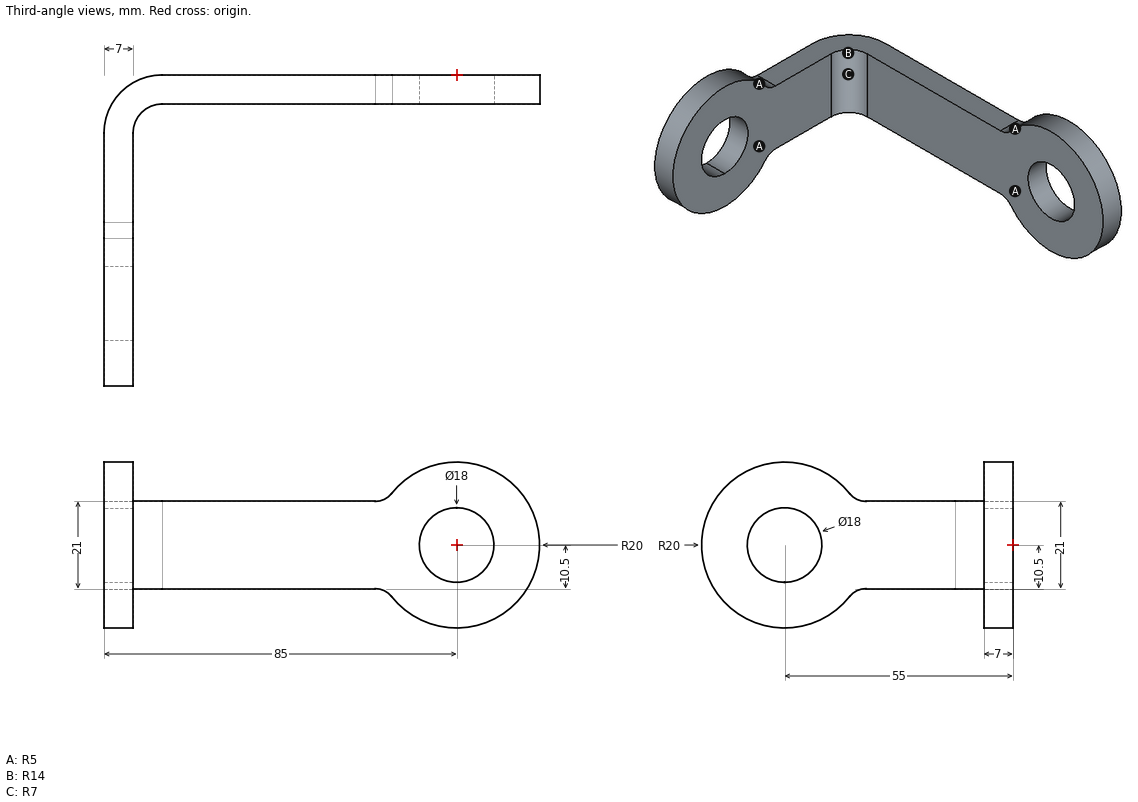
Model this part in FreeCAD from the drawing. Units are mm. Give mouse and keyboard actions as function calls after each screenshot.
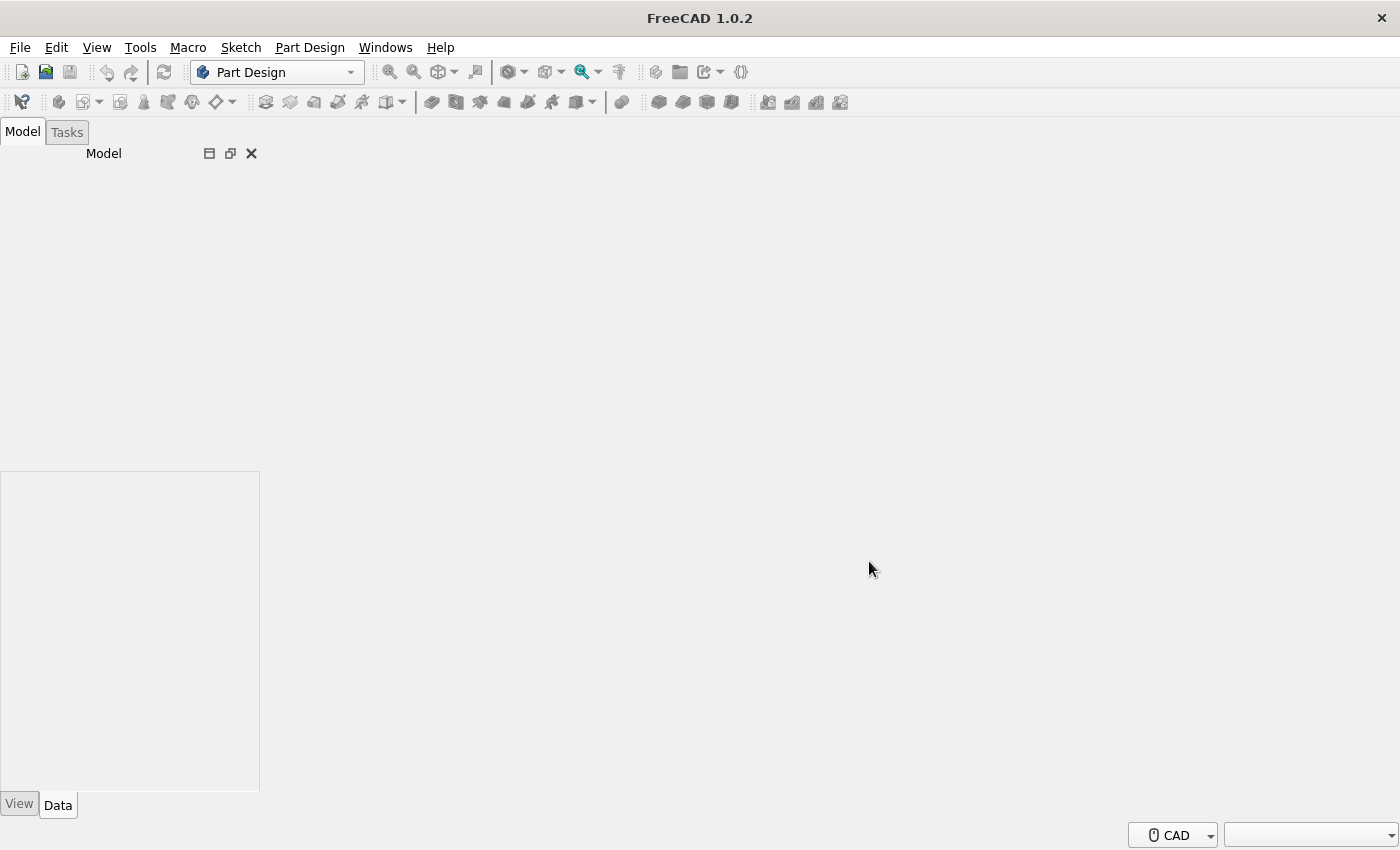
click(22, 72)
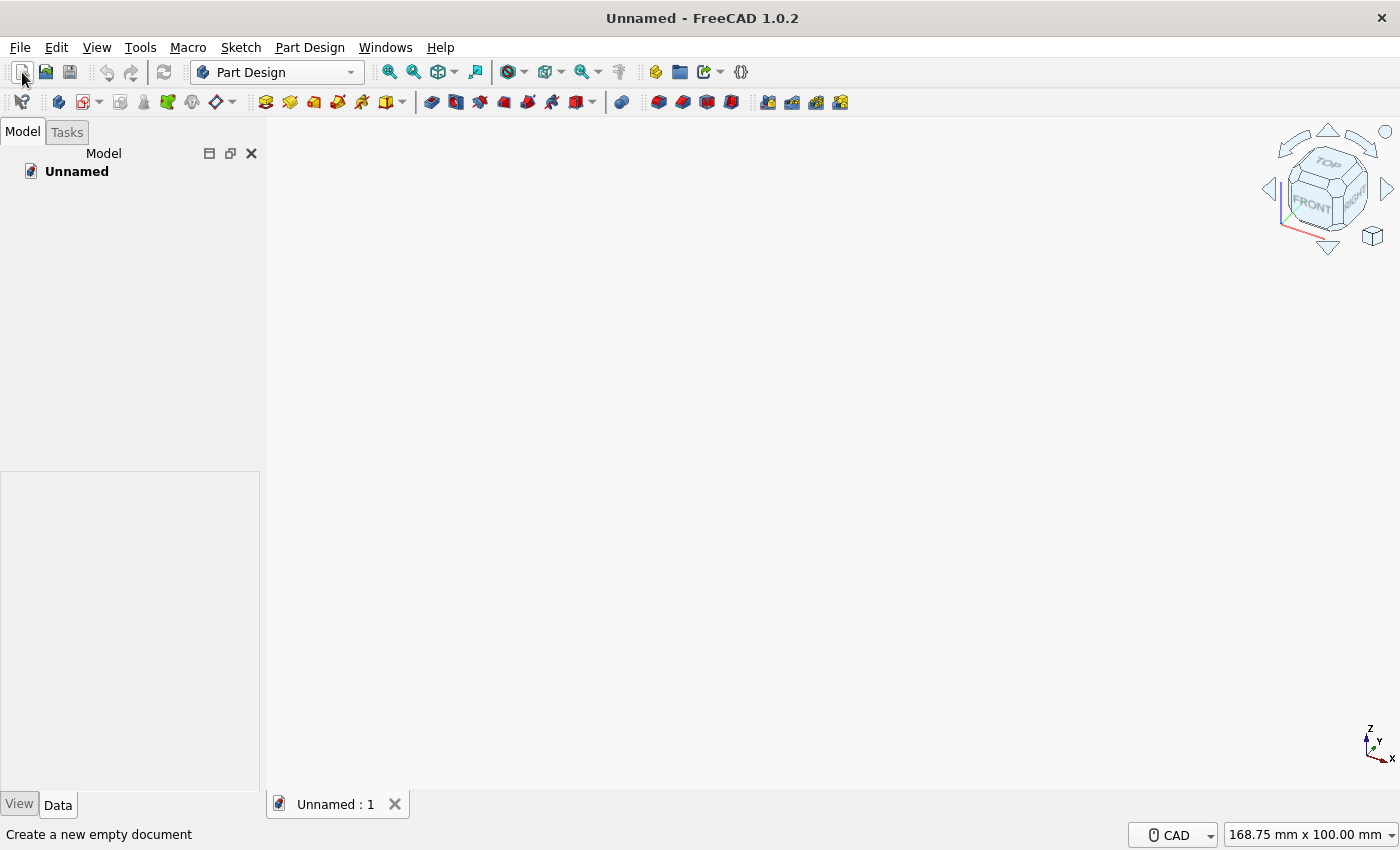
click(84, 102)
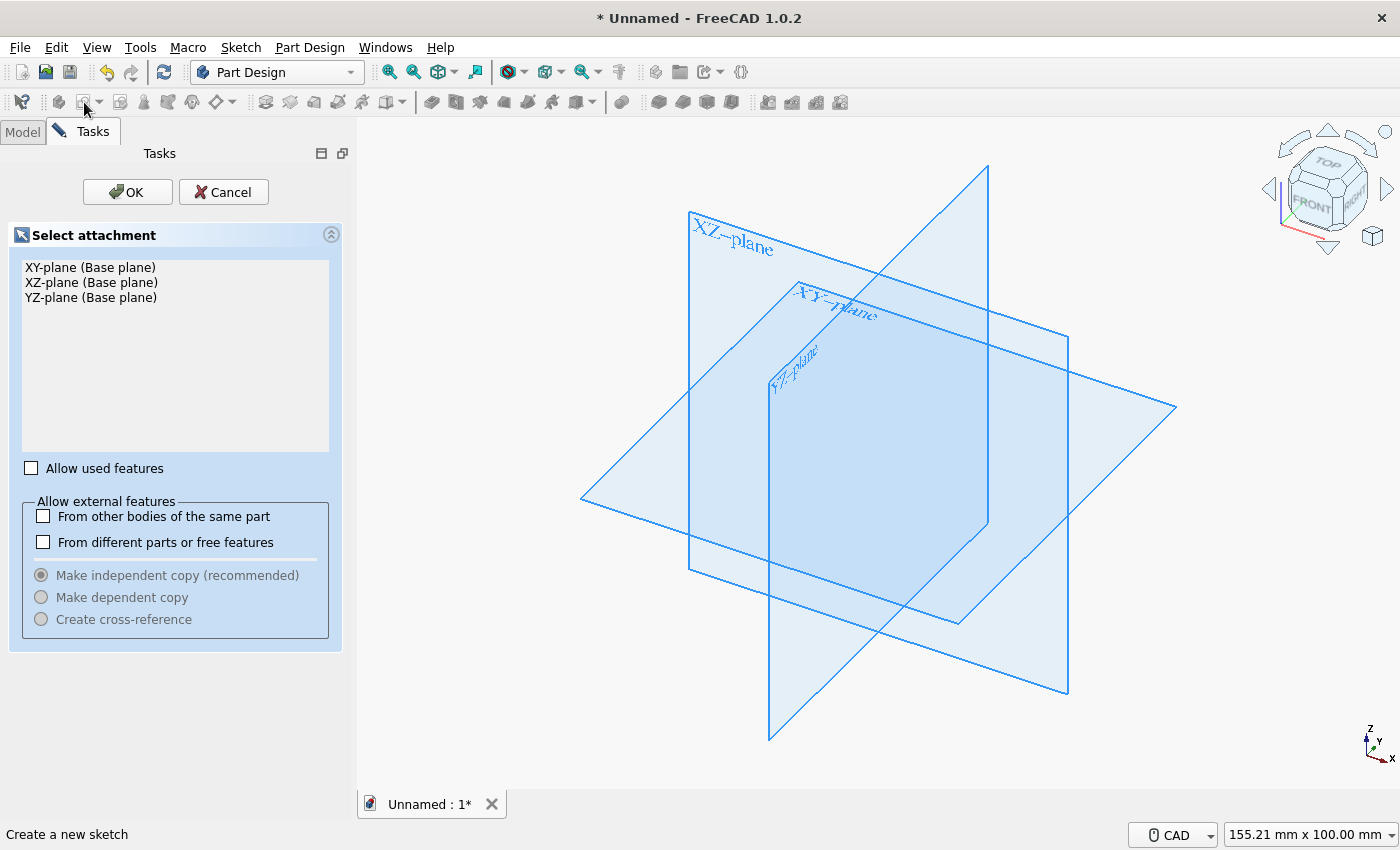
click(82, 282)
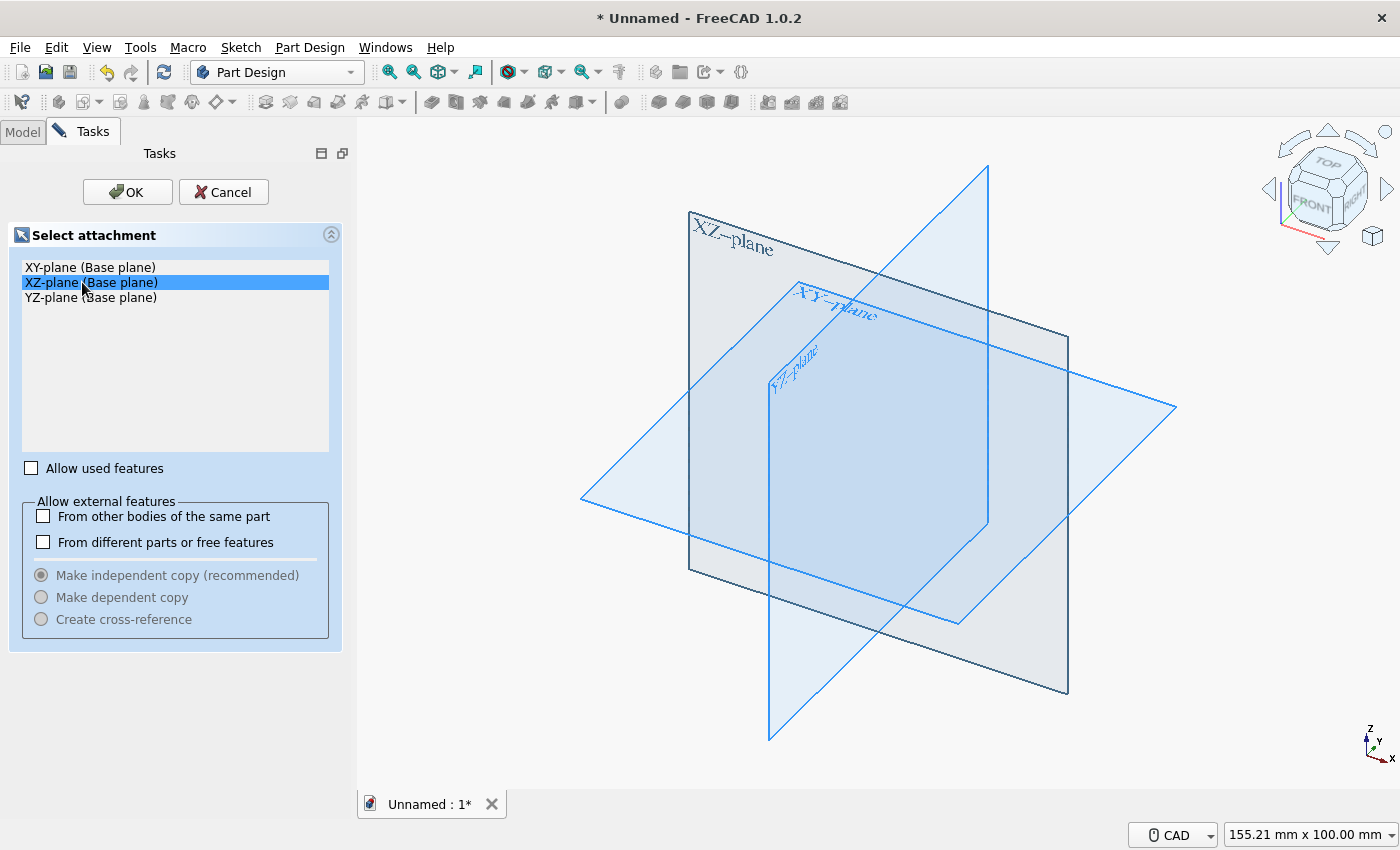
click(128, 192)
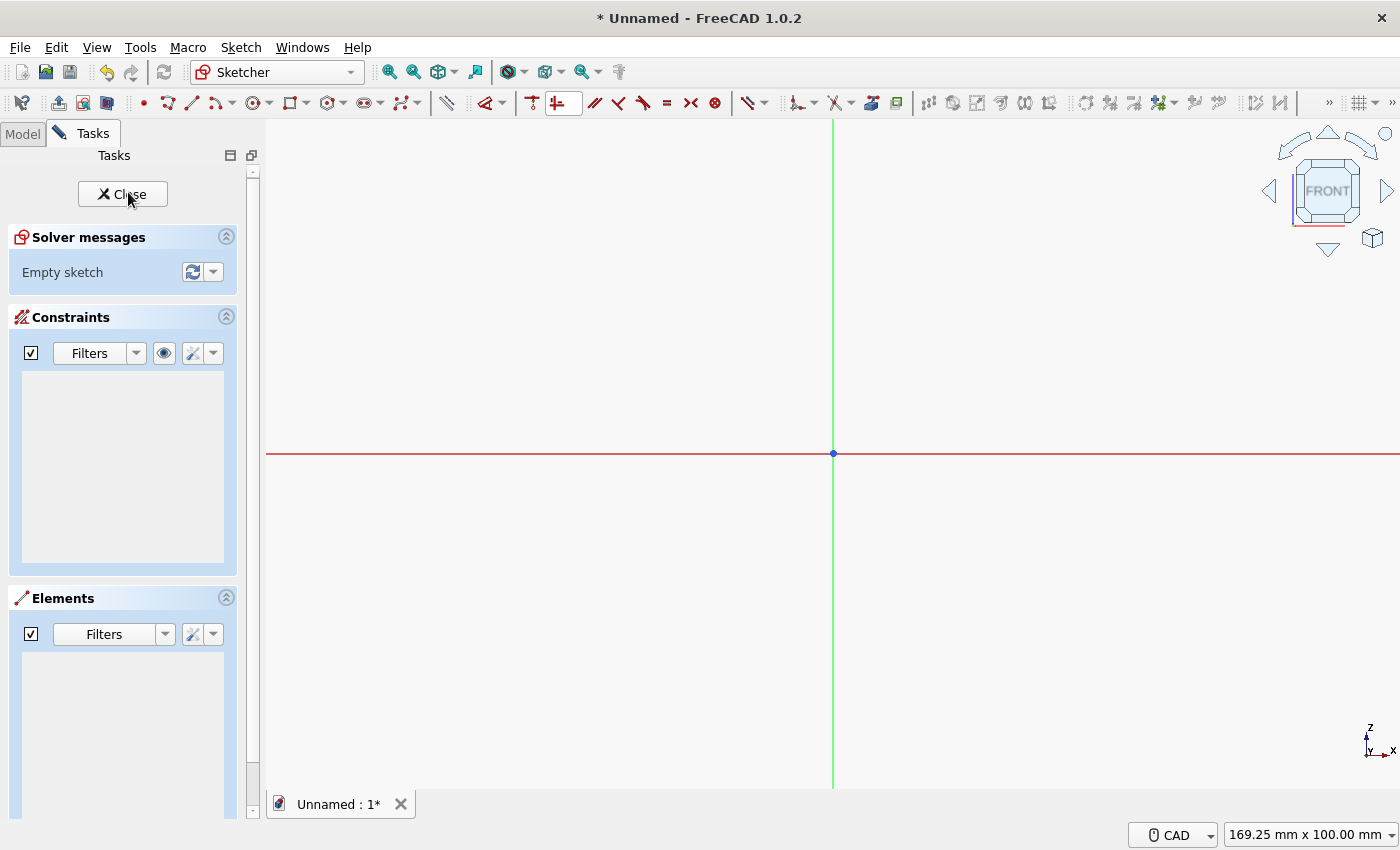
scroll(1235, 454, down, 1)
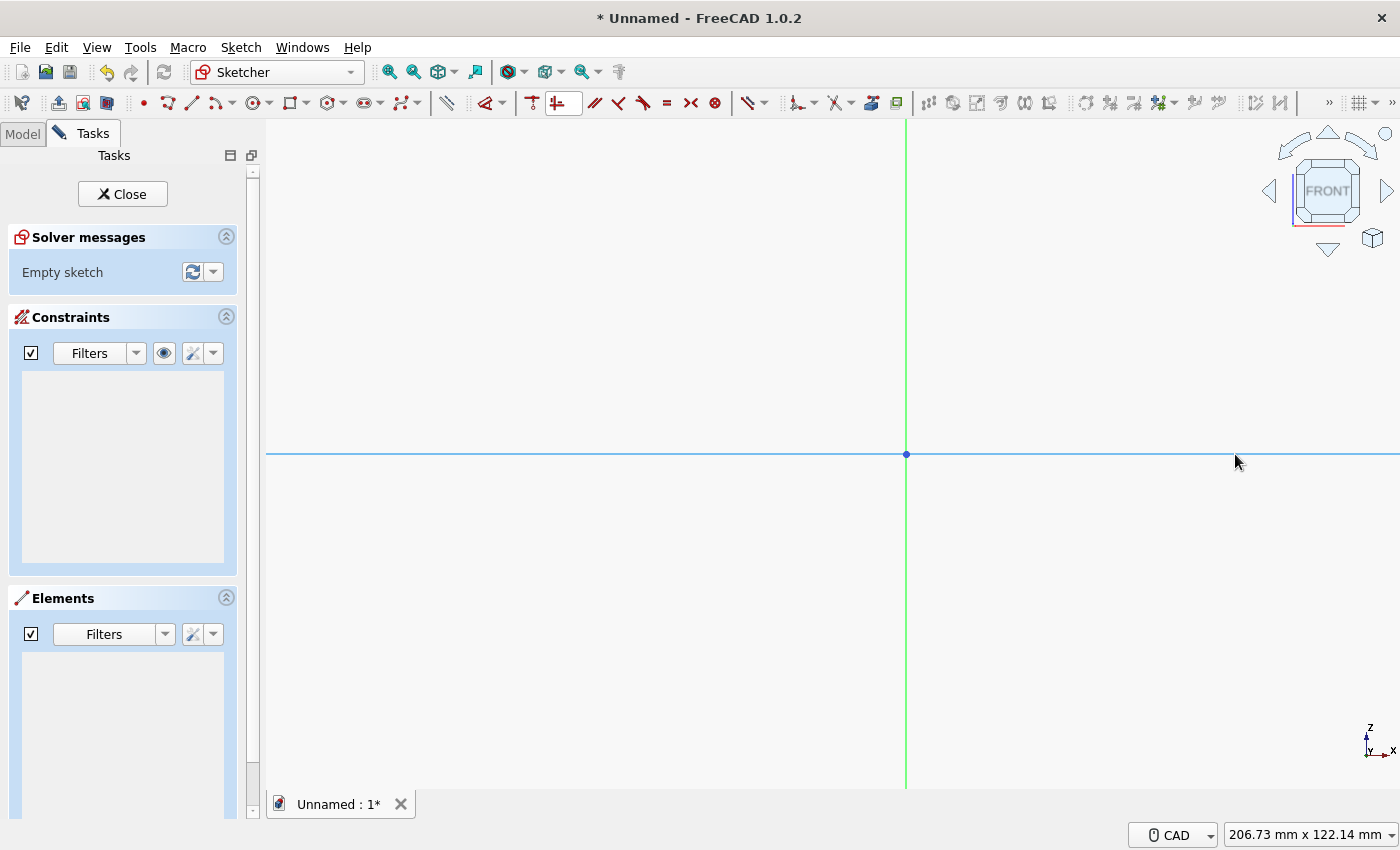
click(168, 104)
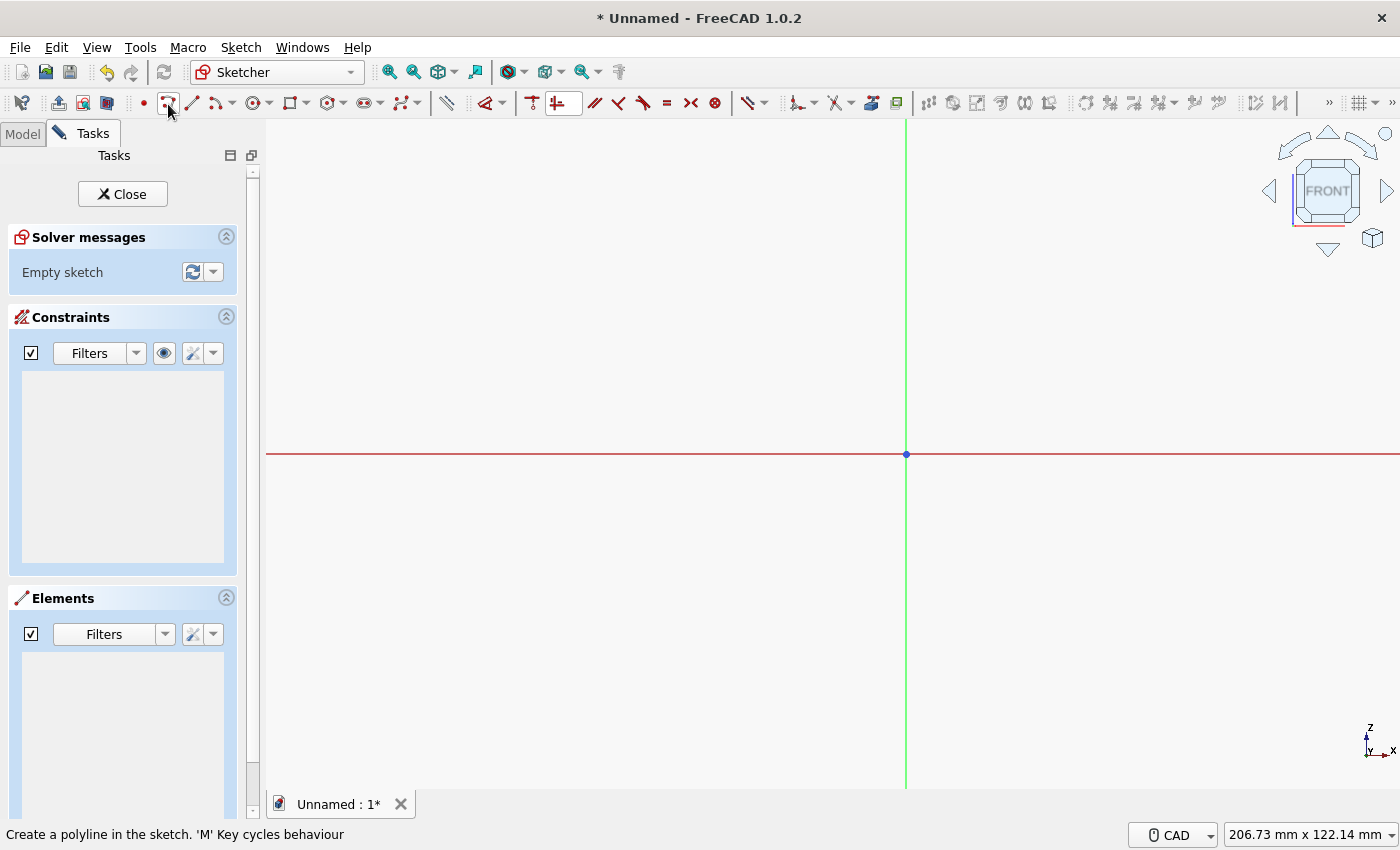
click(813, 512)
click(440, 512)
click(440, 396)
click(813, 396)
right_click(813, 396)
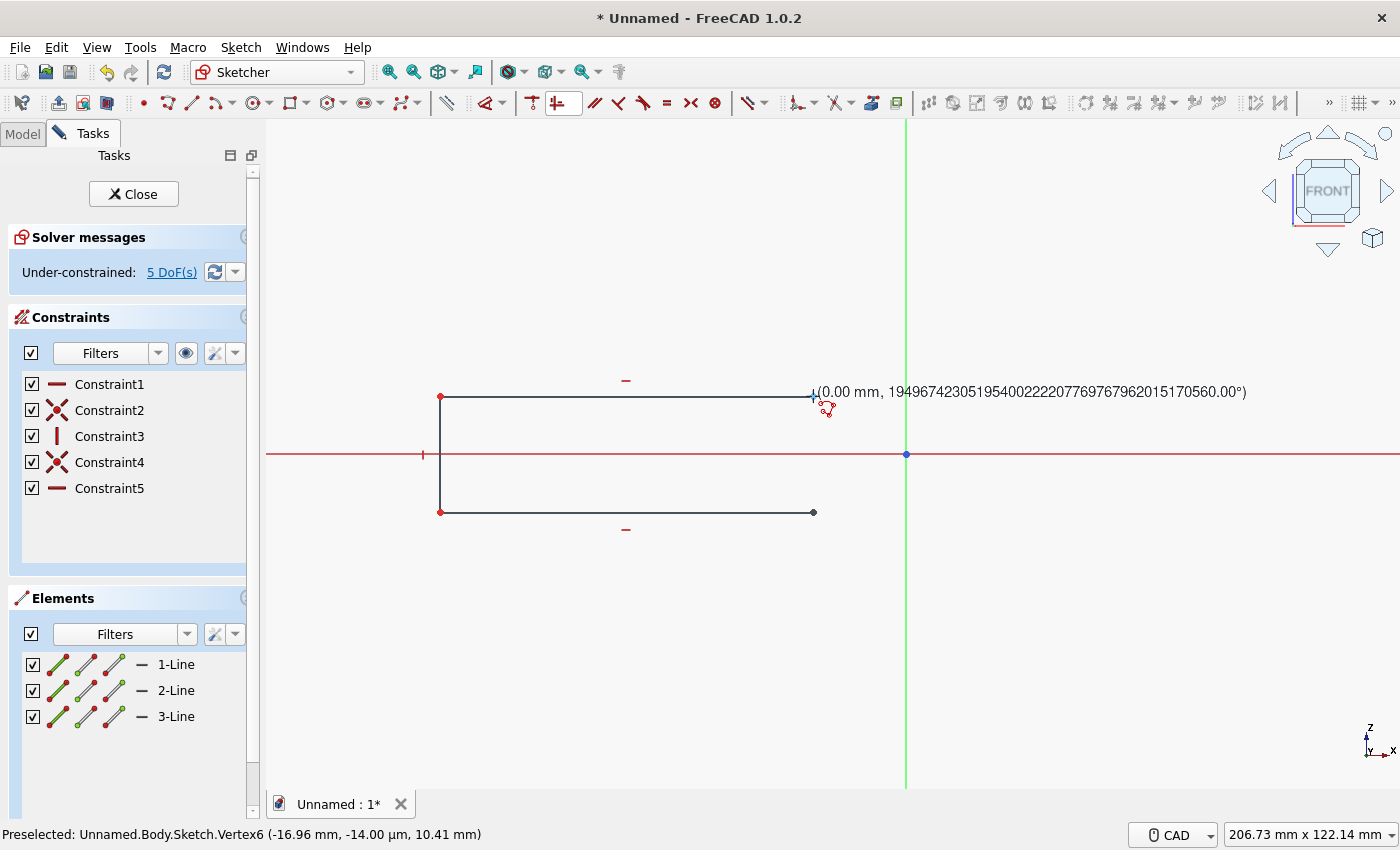
click(234, 104)